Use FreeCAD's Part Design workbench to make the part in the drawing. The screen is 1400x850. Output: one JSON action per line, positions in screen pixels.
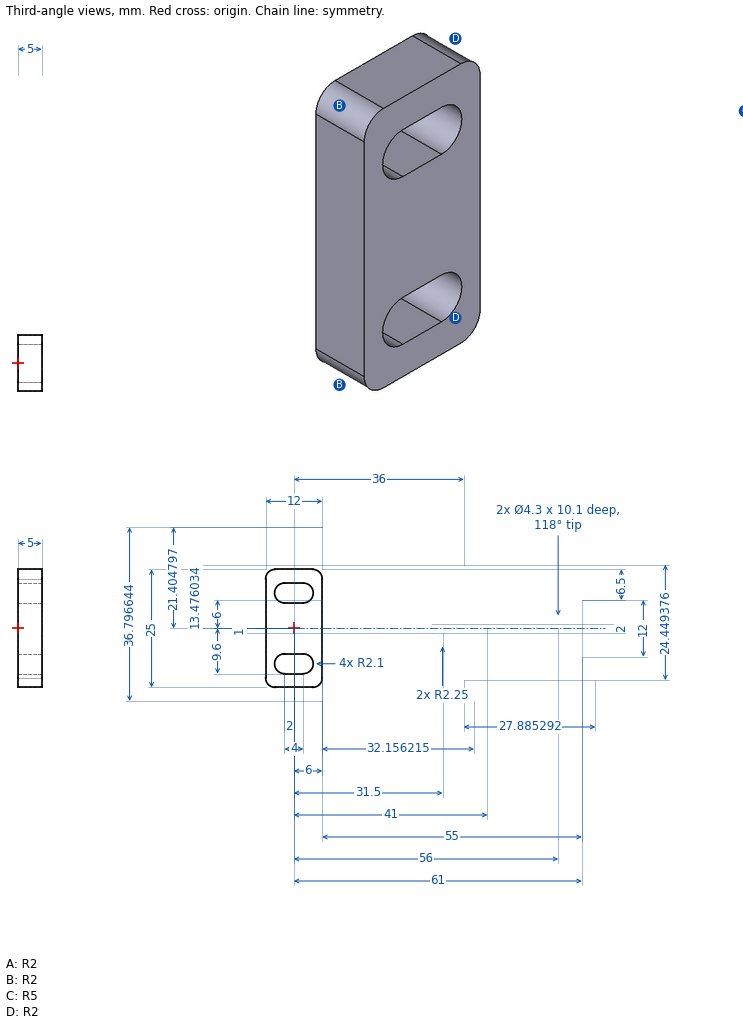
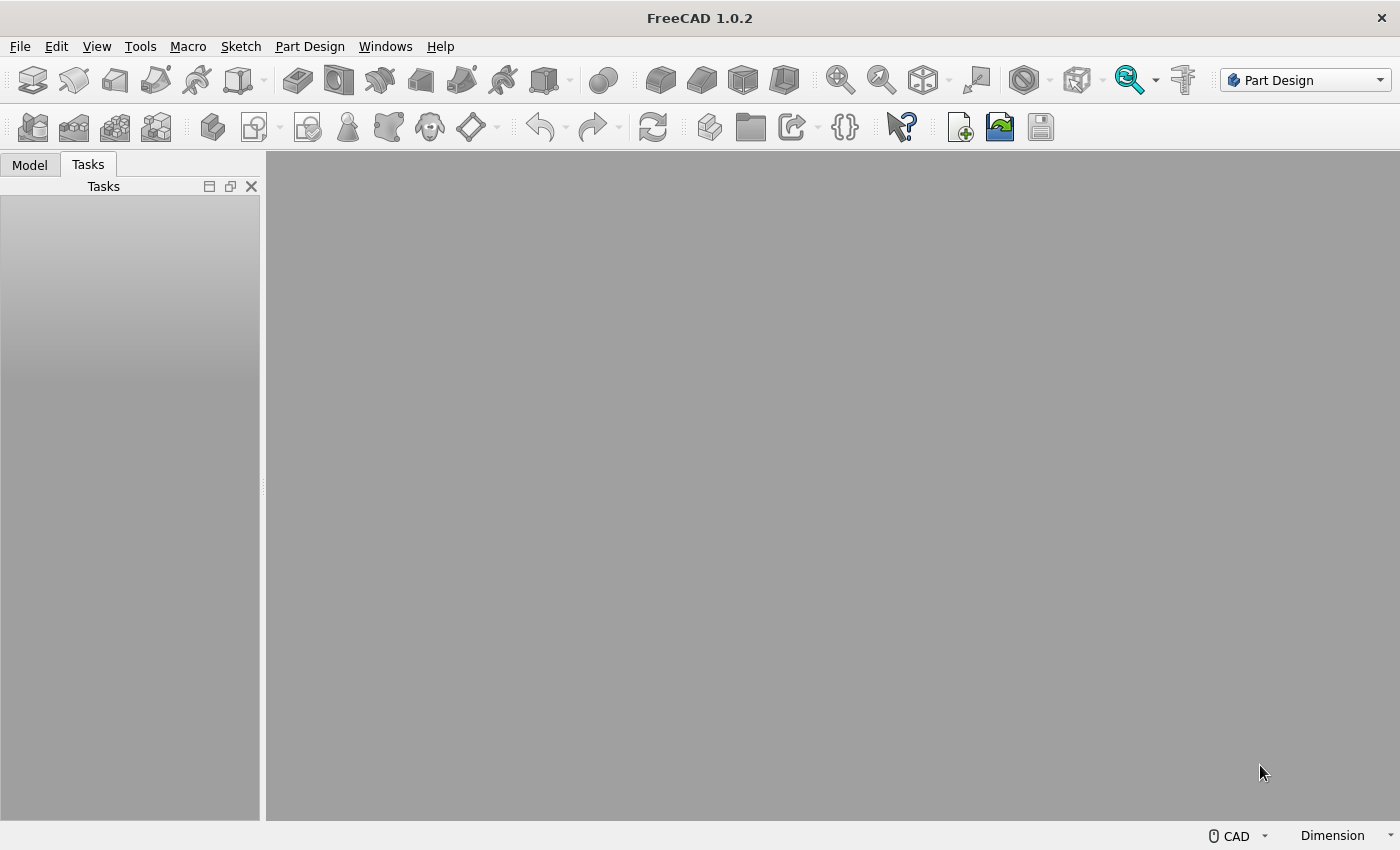
{"action": "key", "text": "ctrl+n"}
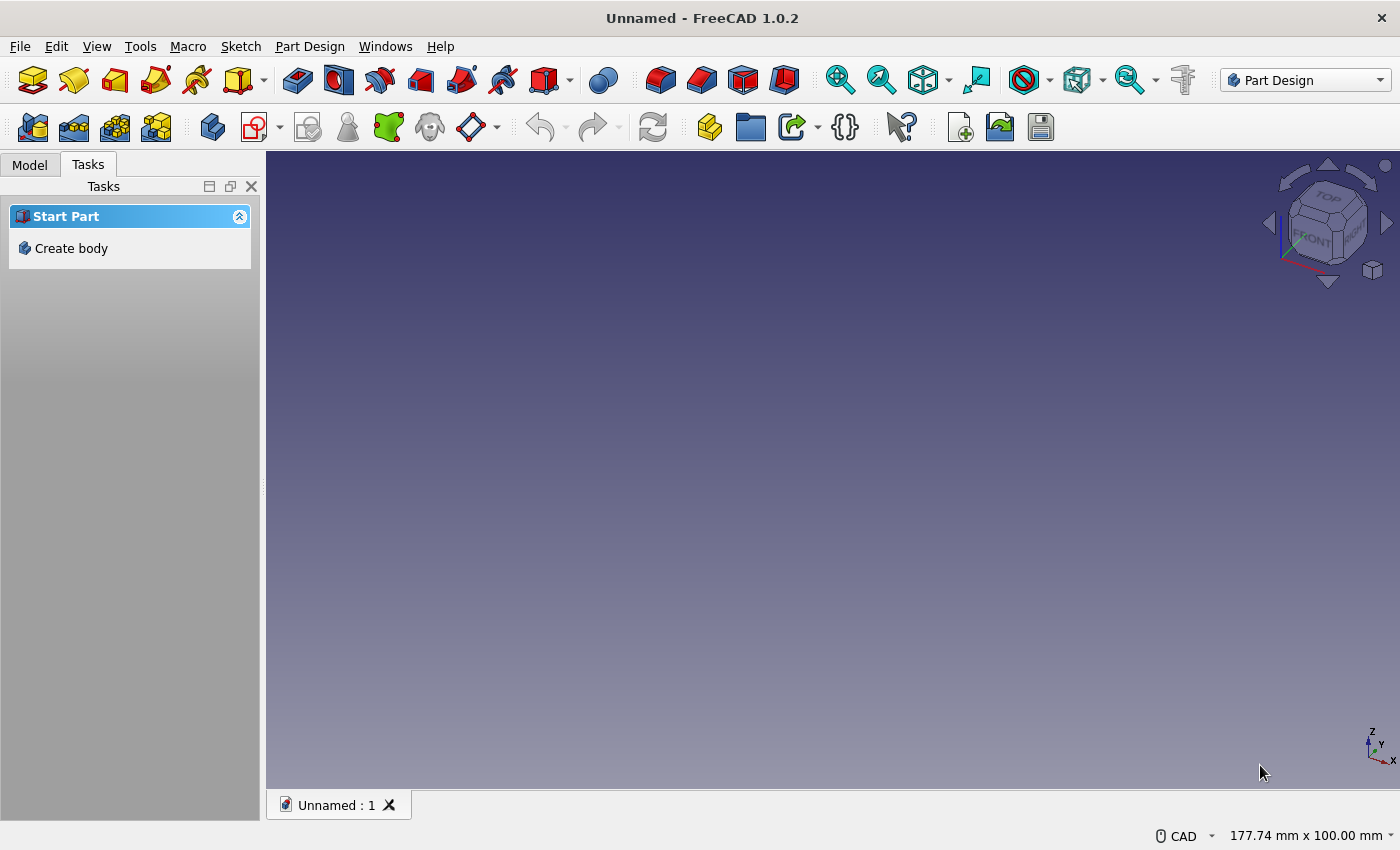
{"action": "left_click", "coordinate": [254, 128]}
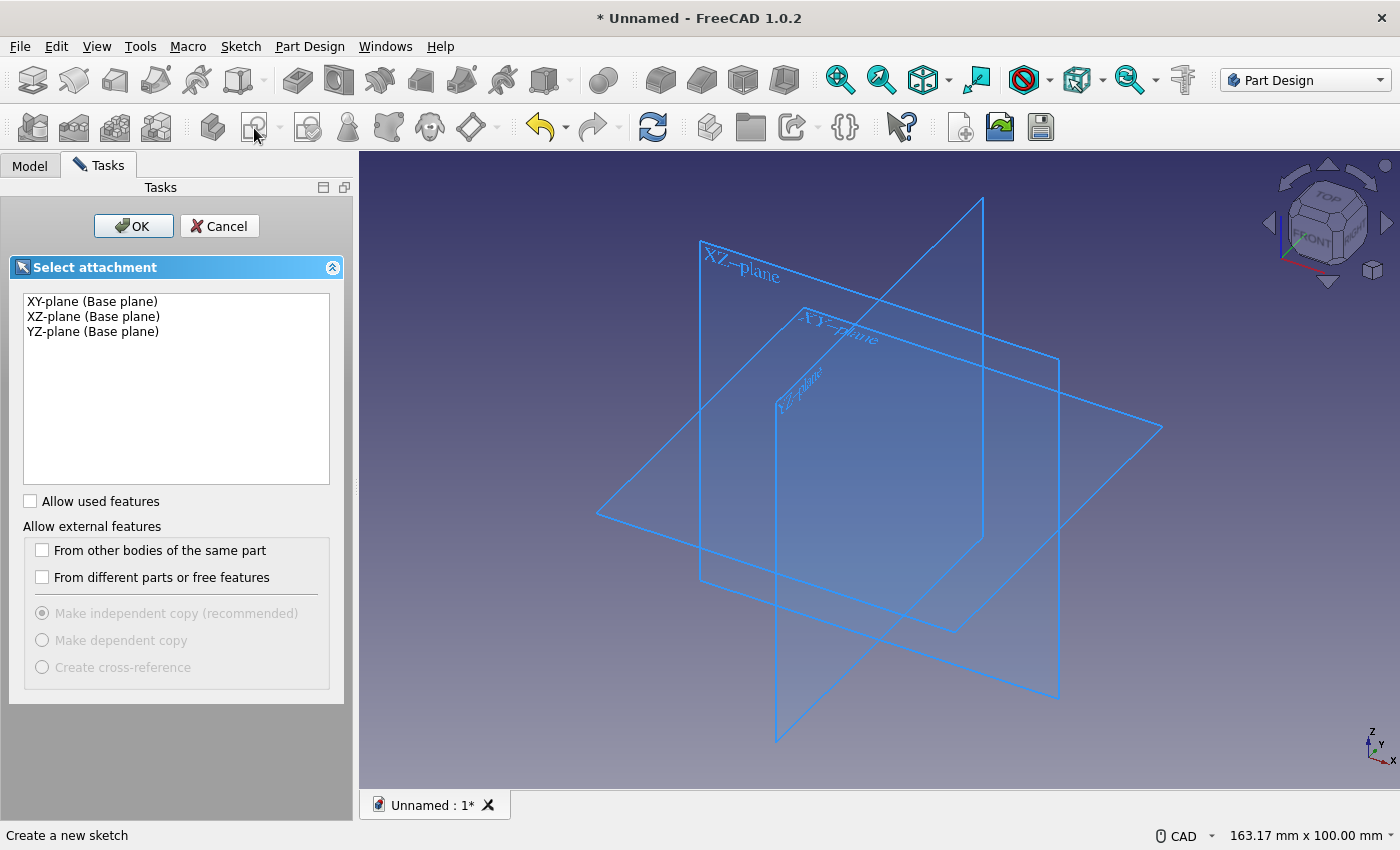
{"action": "left_click", "coordinate": [84, 332]}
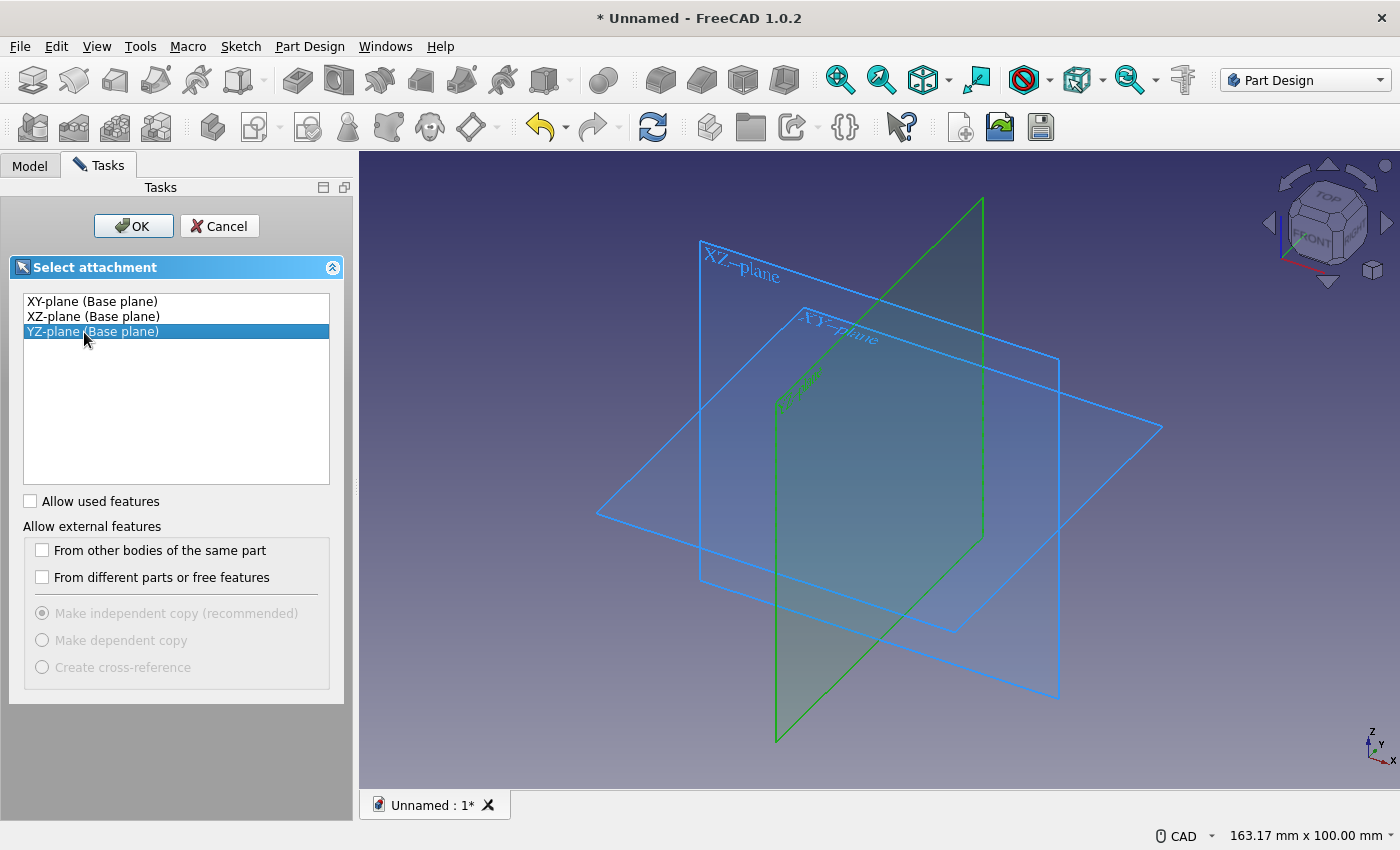
{"action": "left_click", "coordinate": [134, 226]}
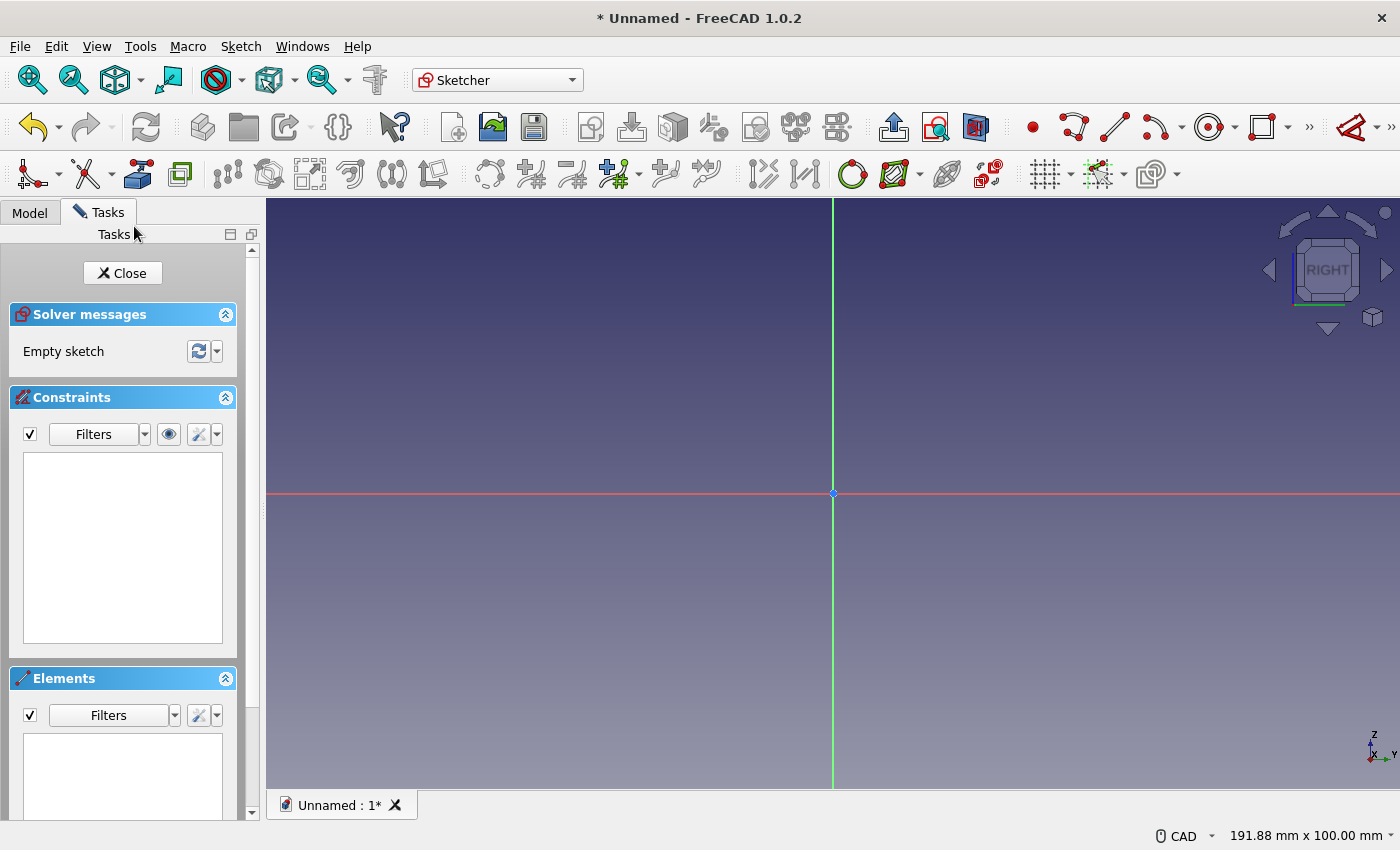
{"action": "scroll", "coordinate": [1235, 494], "scroll_direction": "up", "scroll_amount": 3}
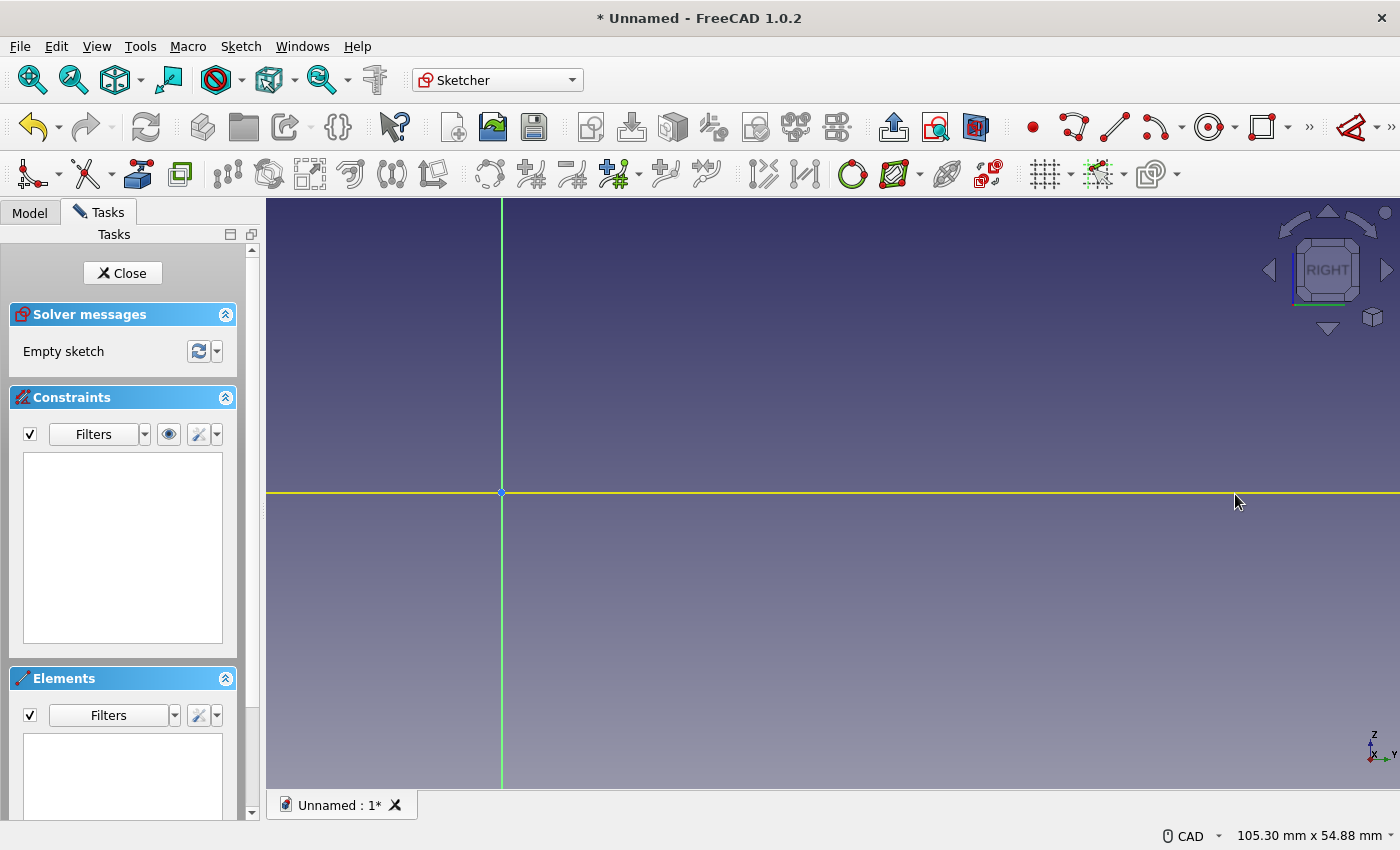
{"action": "left_click", "coordinate": [1074, 128]}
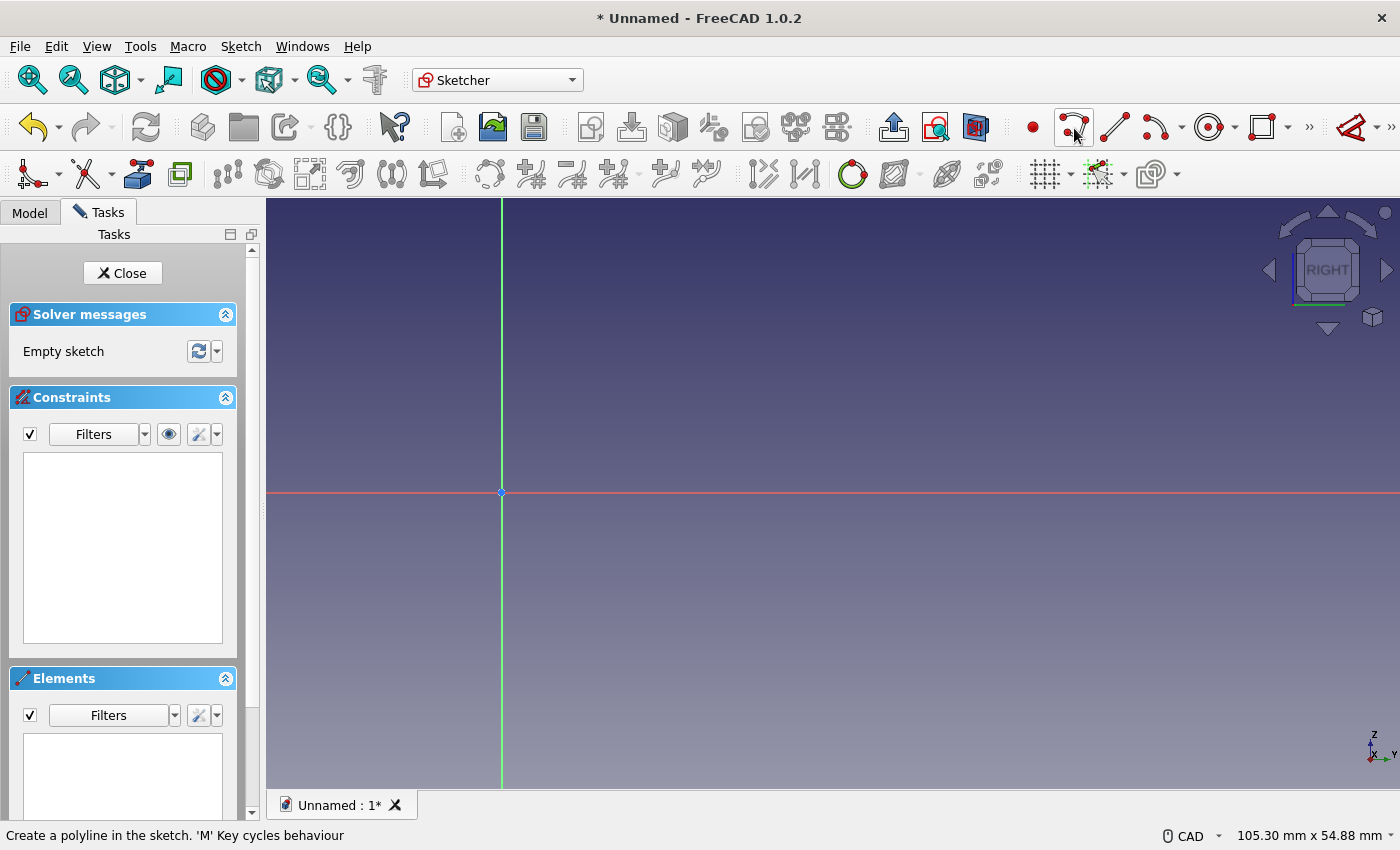
{"action": "left_click", "coordinate": [566, 428]}
{"action": "left_click", "coordinate": [566, 358]}
{"action": "left_click", "coordinate": [437, 358]}
{"action": "left_click", "coordinate": [437, 627]}
{"action": "left_click", "coordinate": [566, 627]}
{"action": "left_click", "coordinate": [566, 557]}
{"action": "left_click", "coordinate": [1159, 557]}
{"action": "left_click", "coordinate": [1159, 428]}
{"action": "left_click", "coordinate": [566, 429]}
{"action": "key", "text": "Escape"}
{"action": "key", "text": "Escape"}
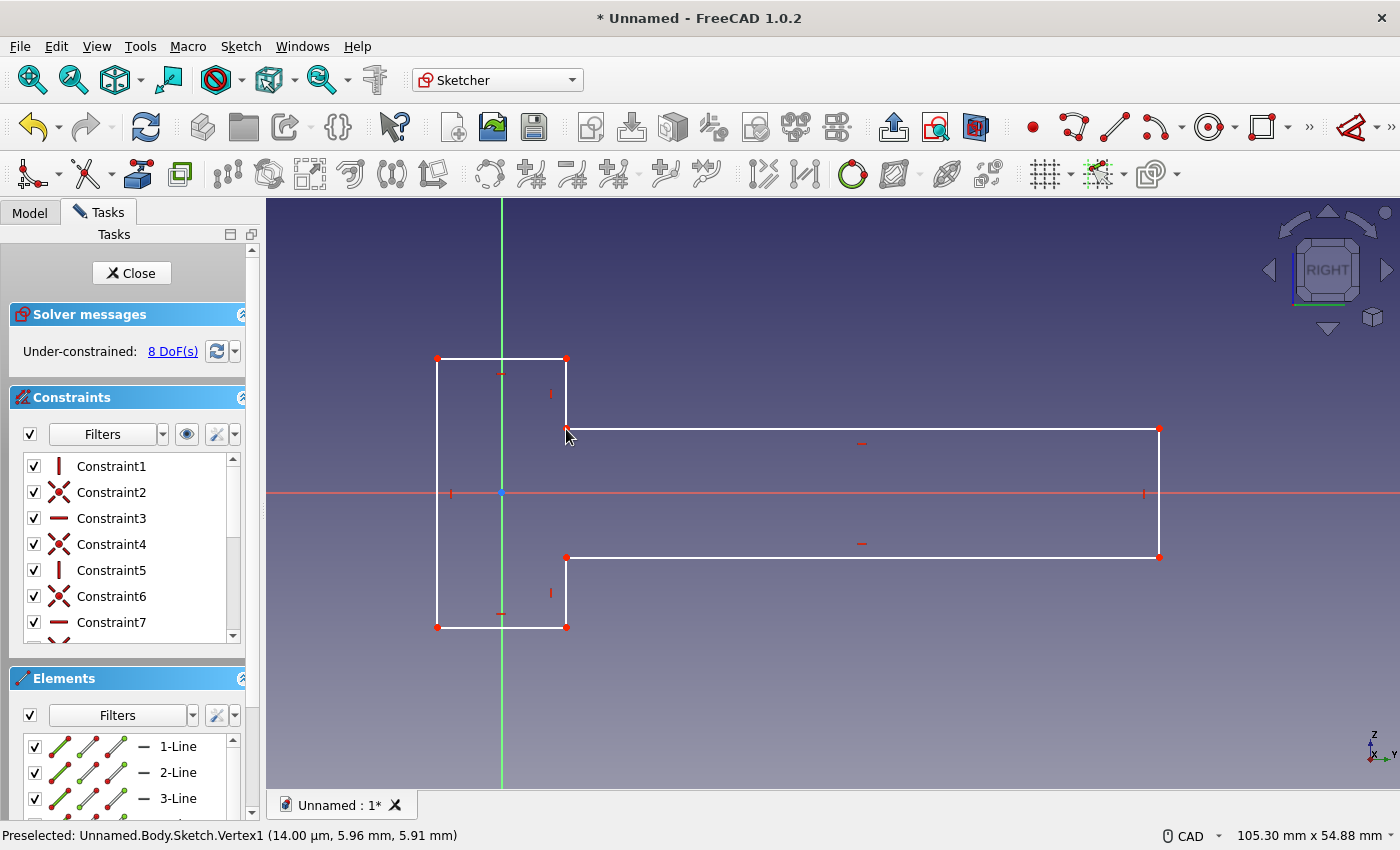
{"action": "left_click", "coordinate": [566, 359]}